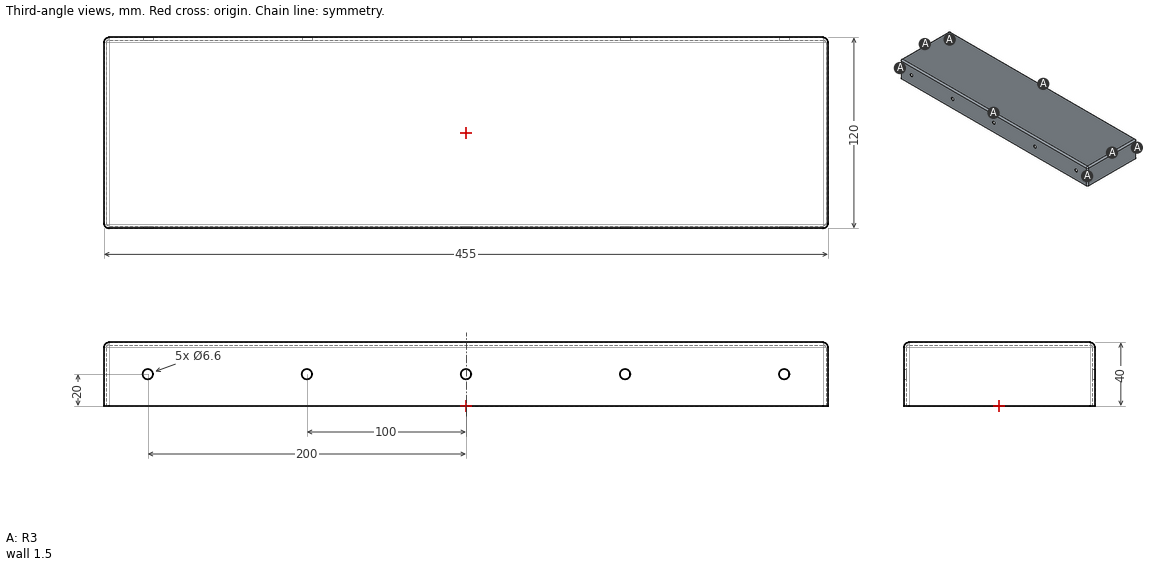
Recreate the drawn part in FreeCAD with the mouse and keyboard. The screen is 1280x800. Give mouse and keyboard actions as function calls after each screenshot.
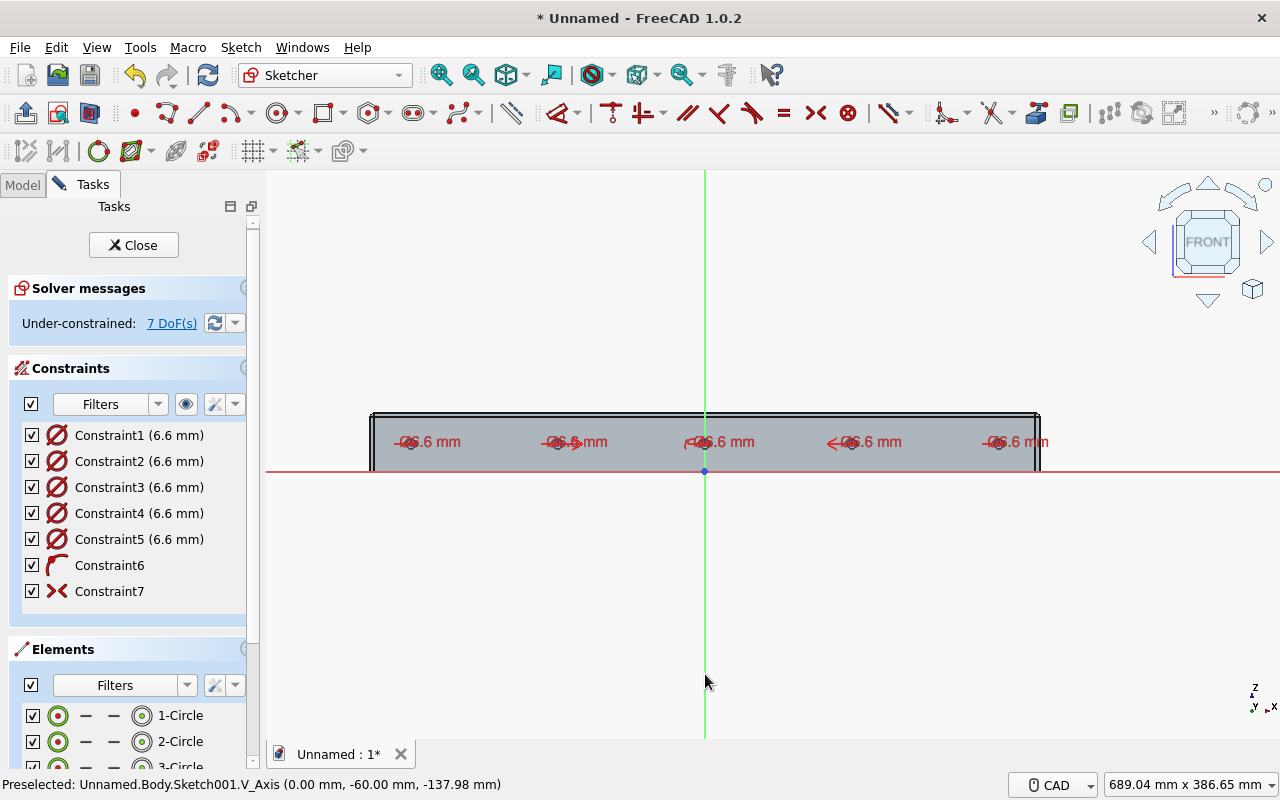
click(411, 444)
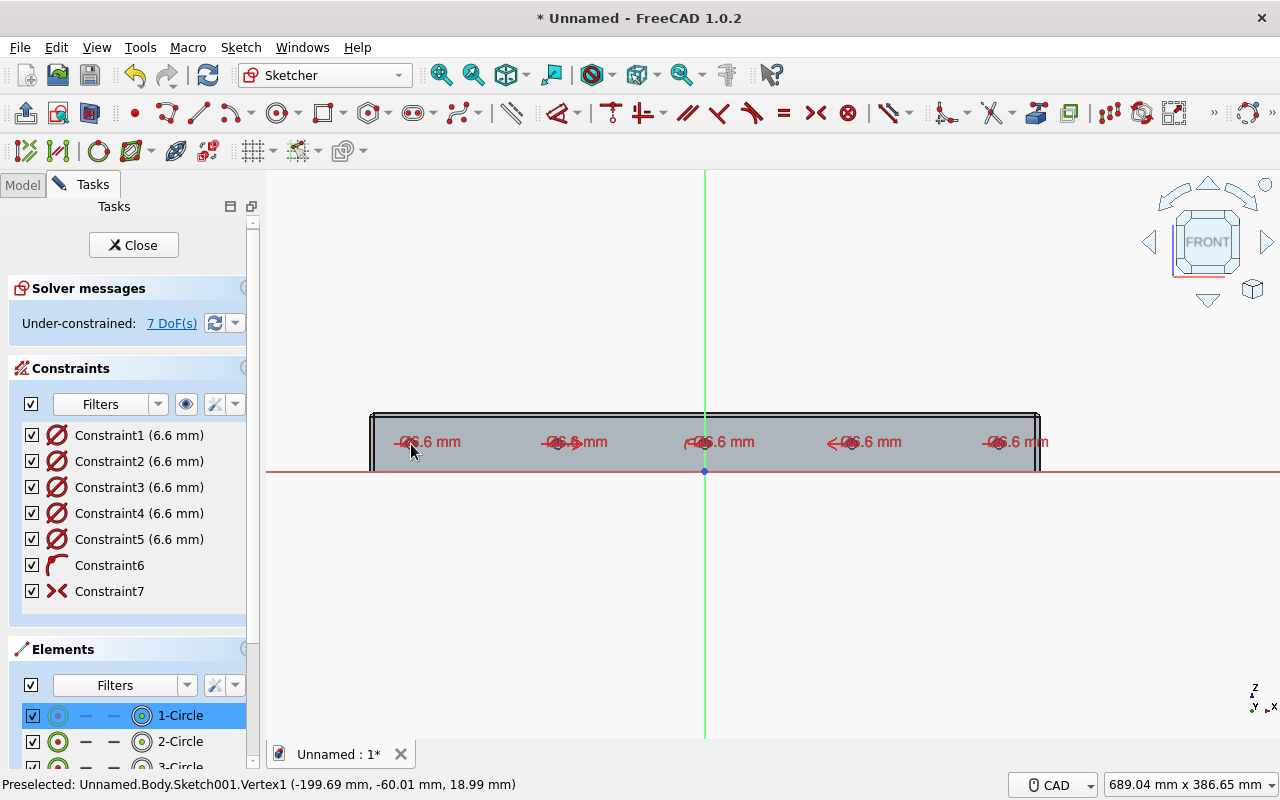
click(999, 444)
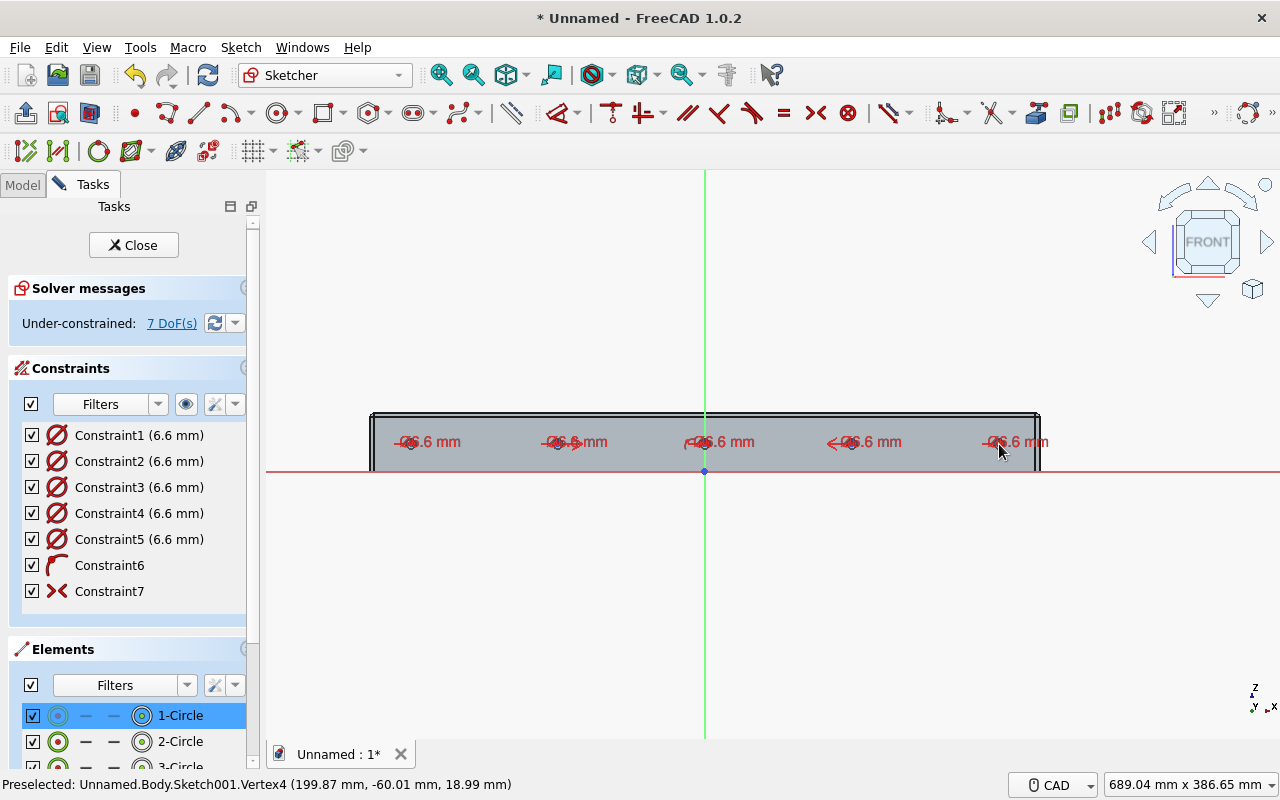
click(705, 674)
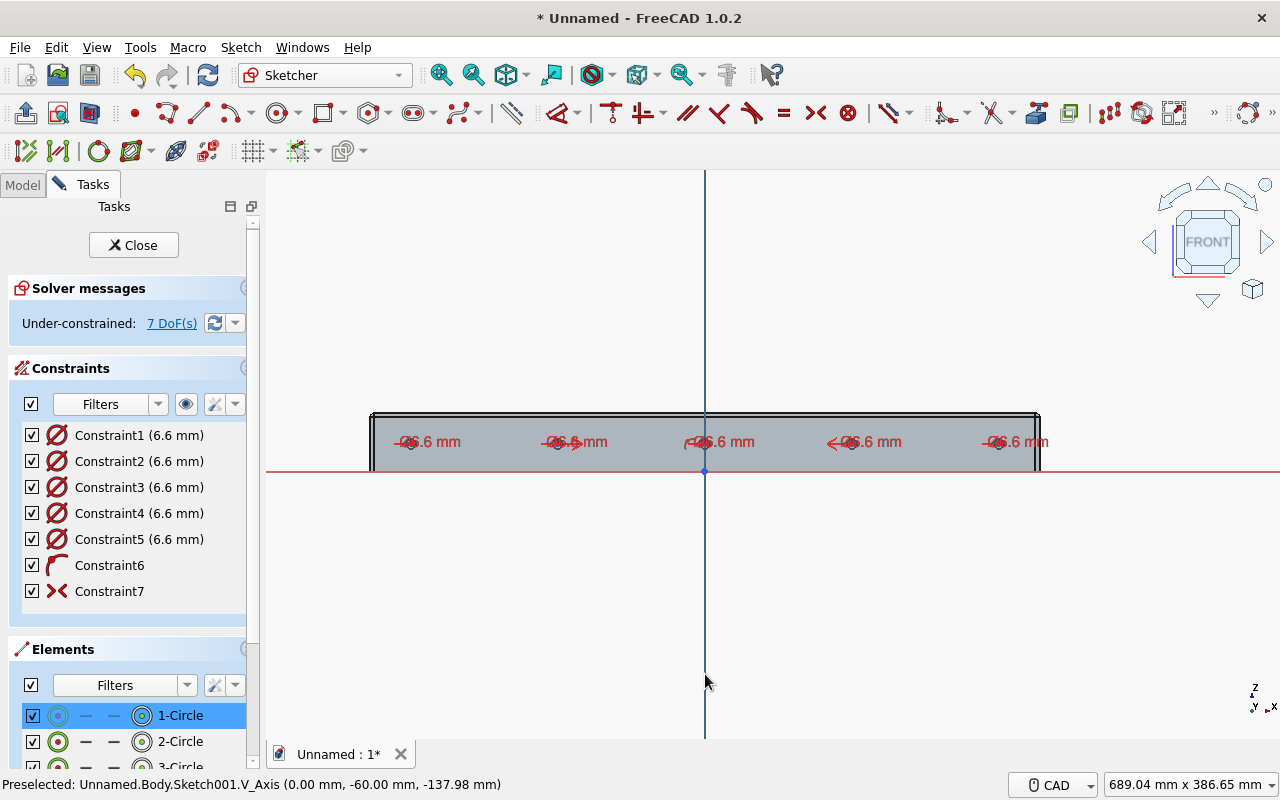
key(s)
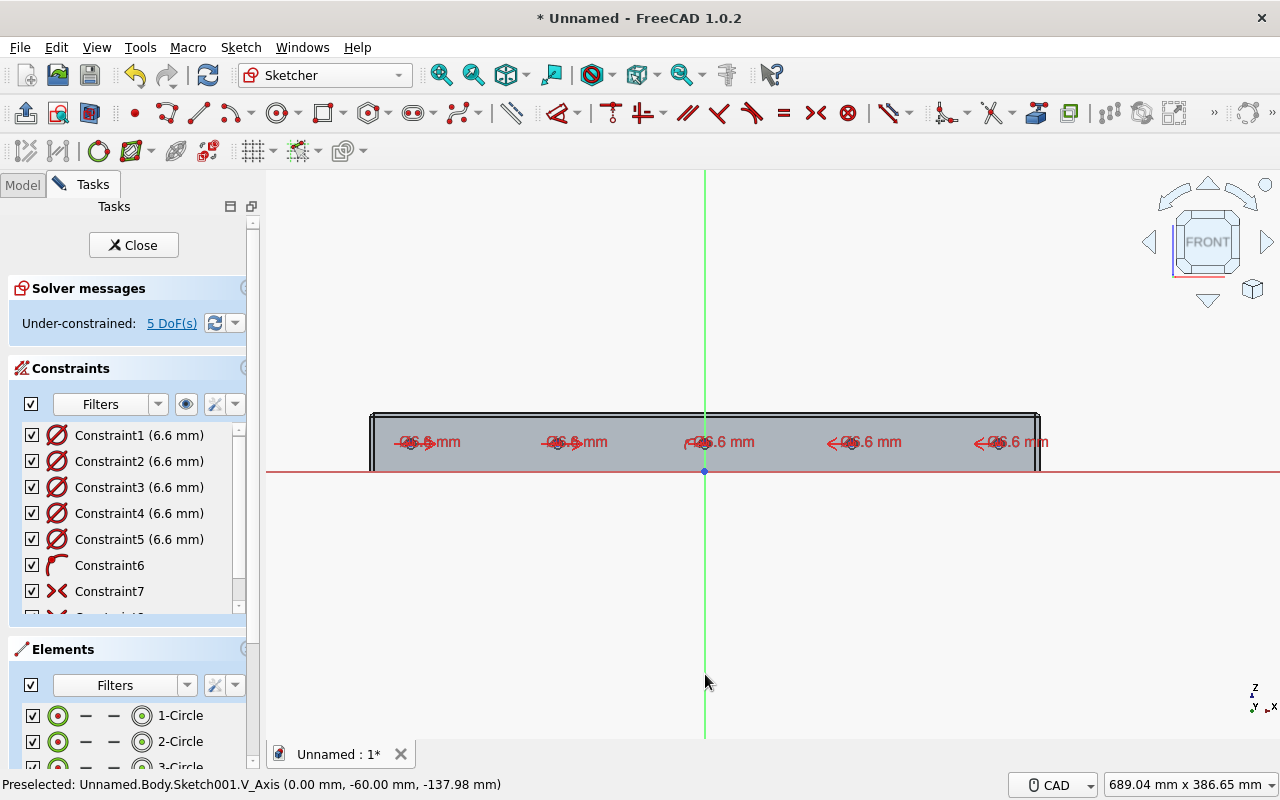
key(d)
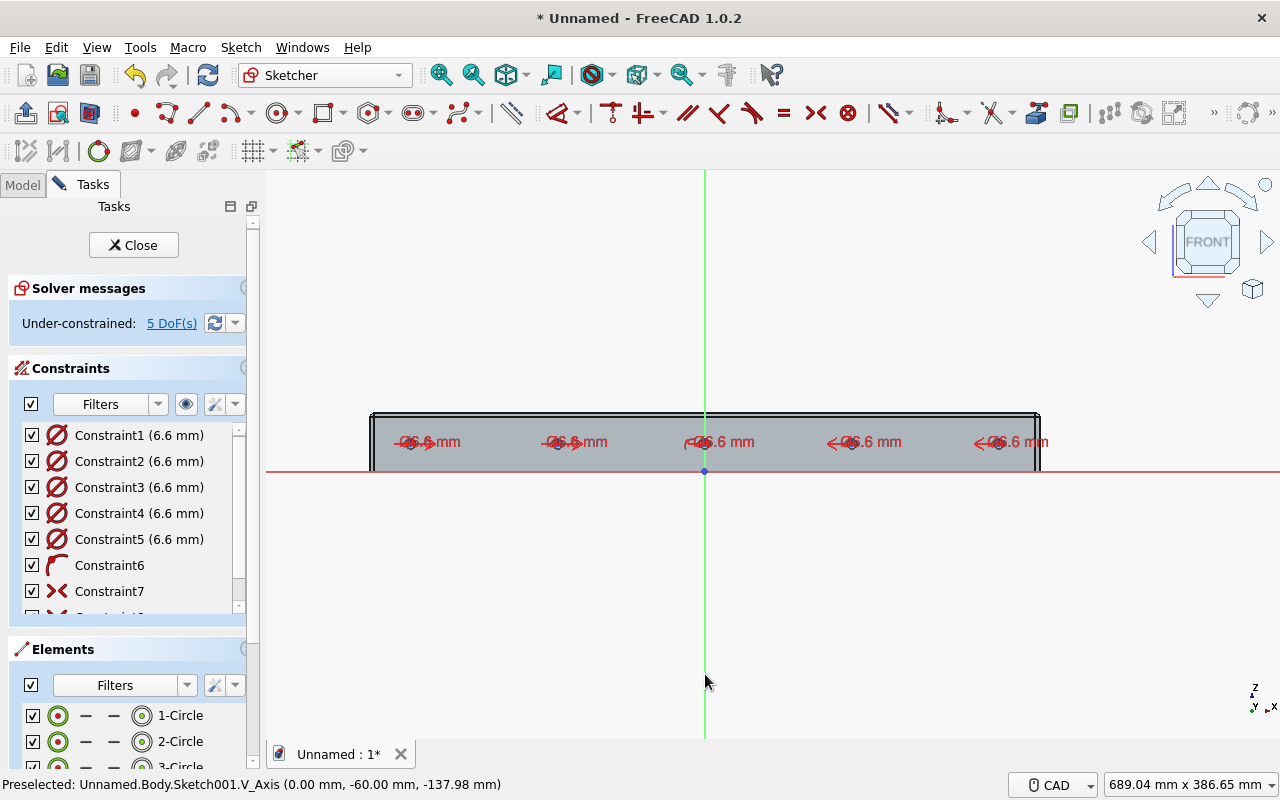
scroll(411, 444, up, 2)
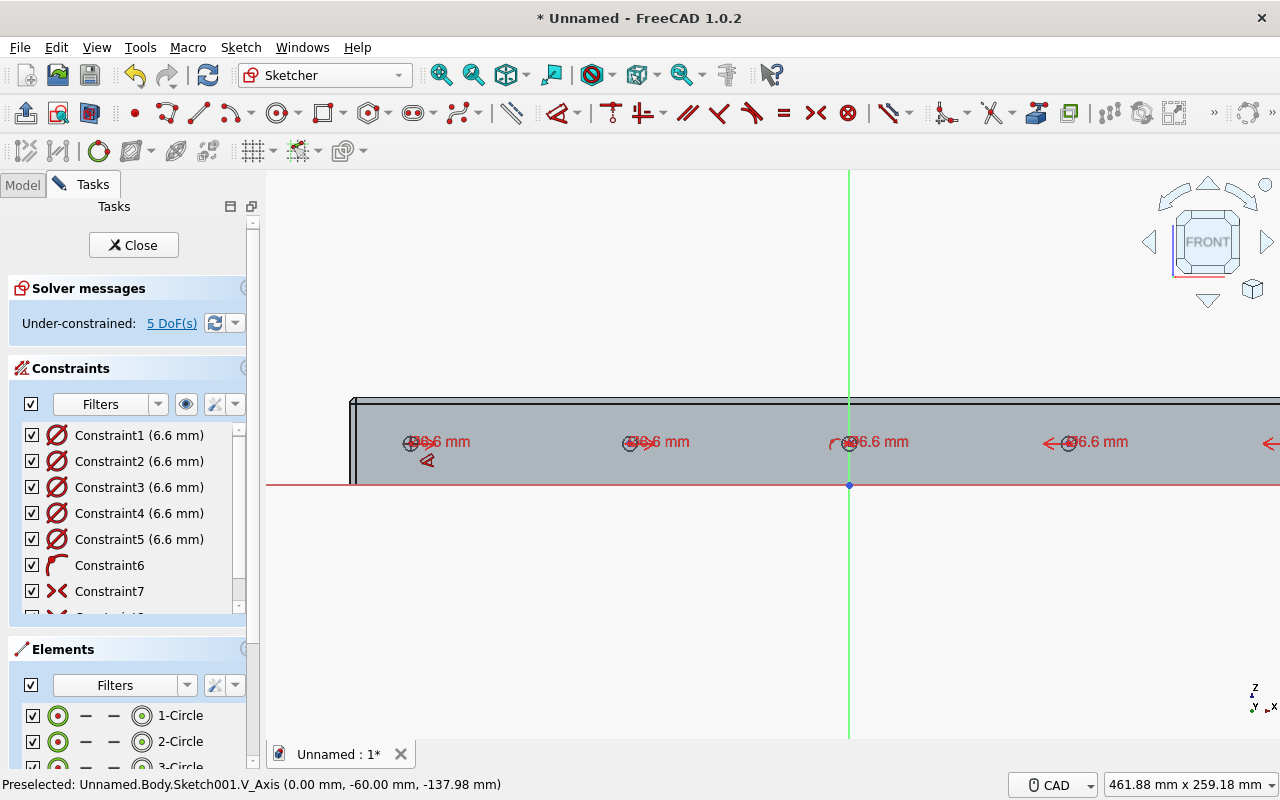
click(411, 444)
click(377, 465)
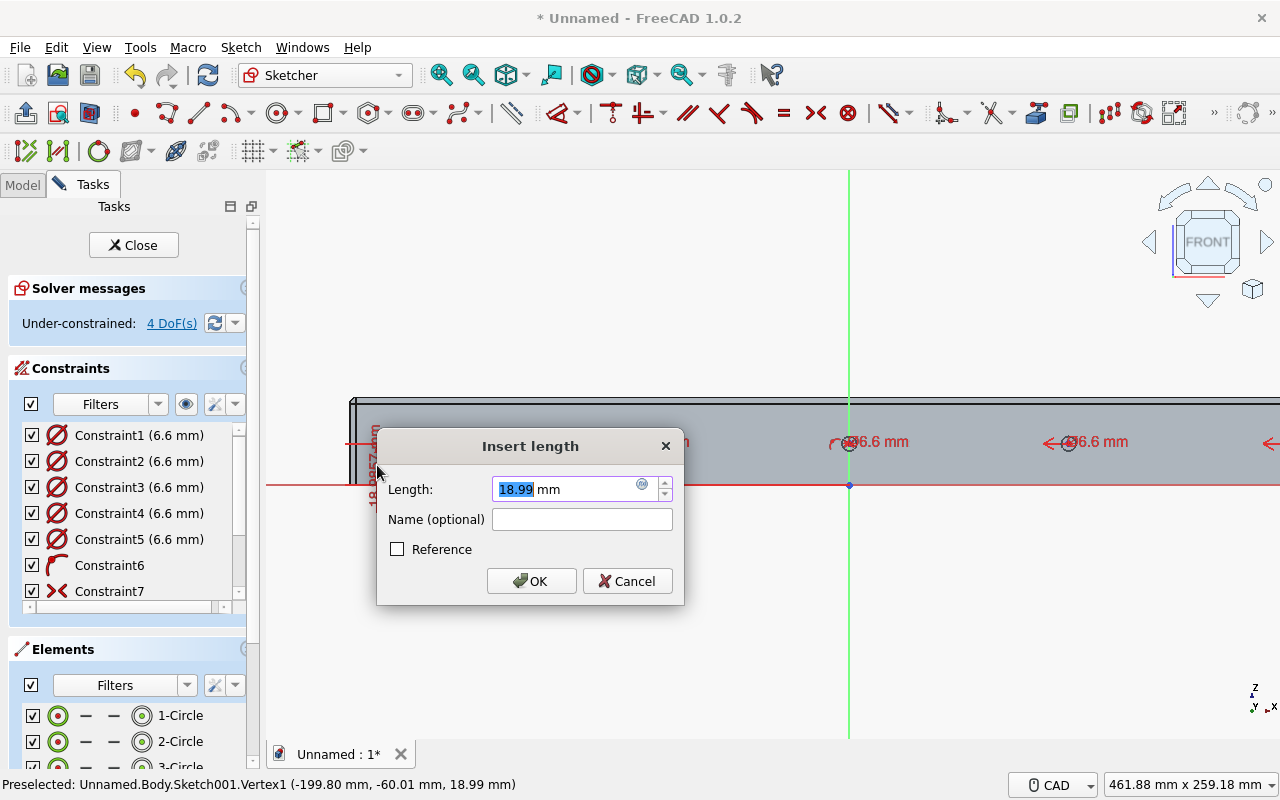
text(20)
key(Return)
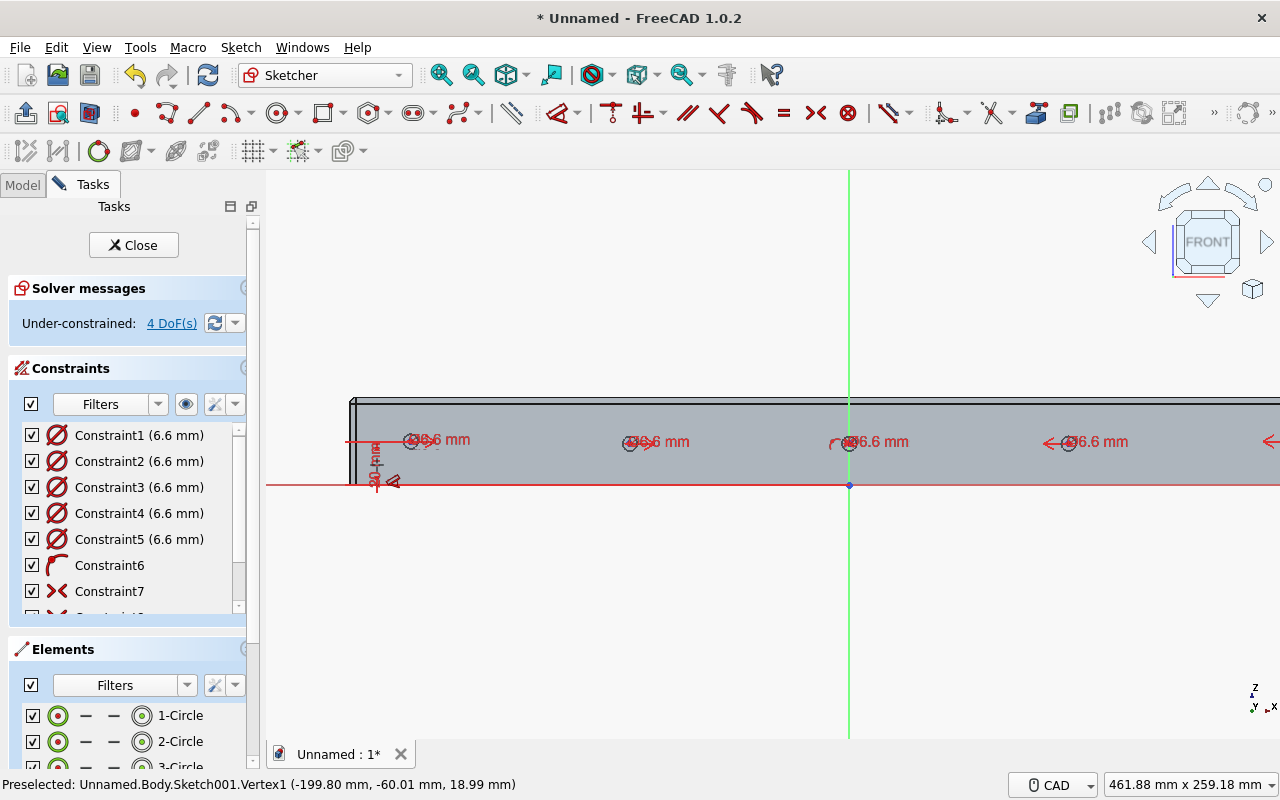
click(630, 444)
click(596, 465)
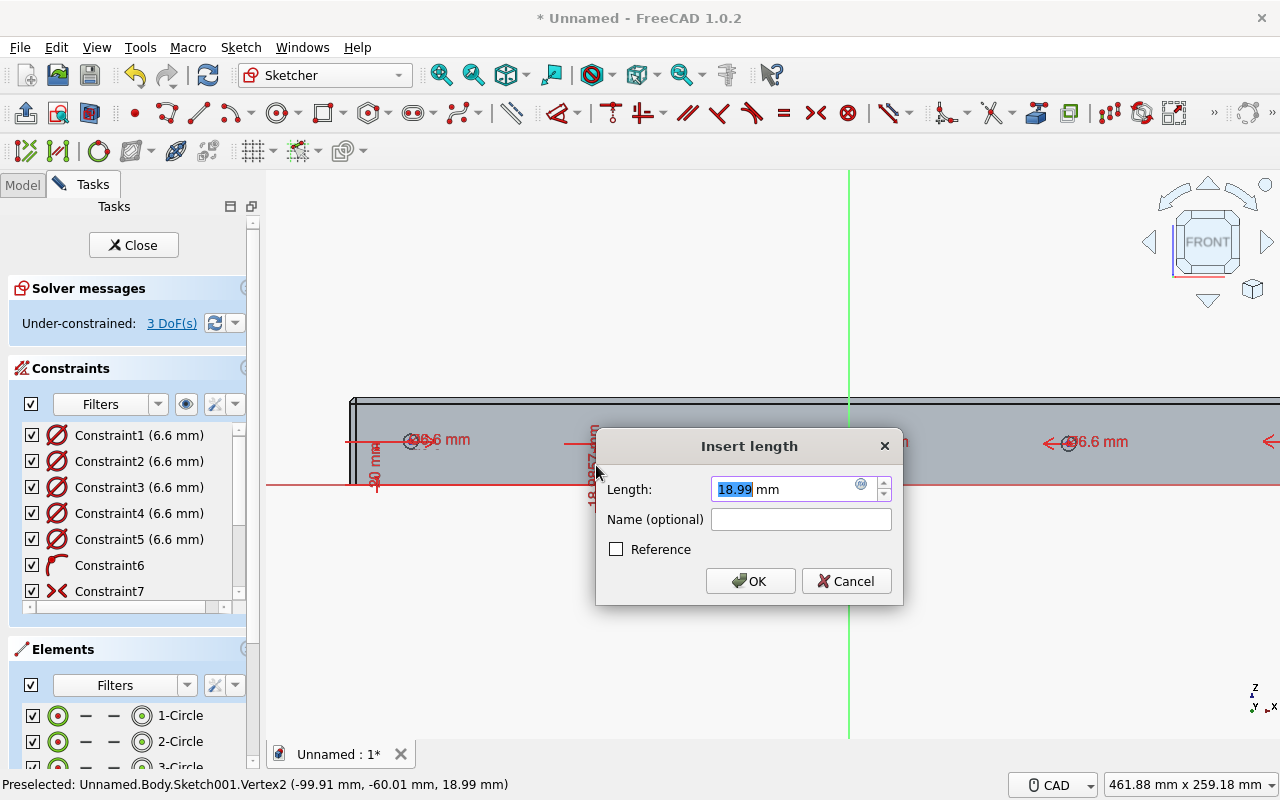
text(20)
key(Return)